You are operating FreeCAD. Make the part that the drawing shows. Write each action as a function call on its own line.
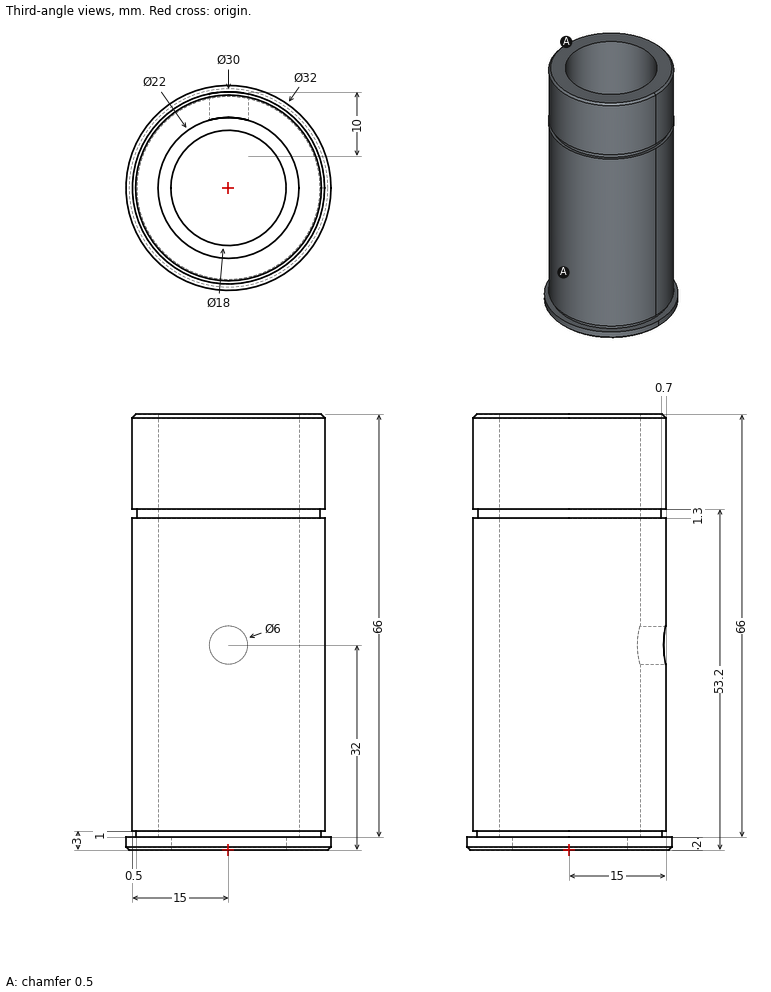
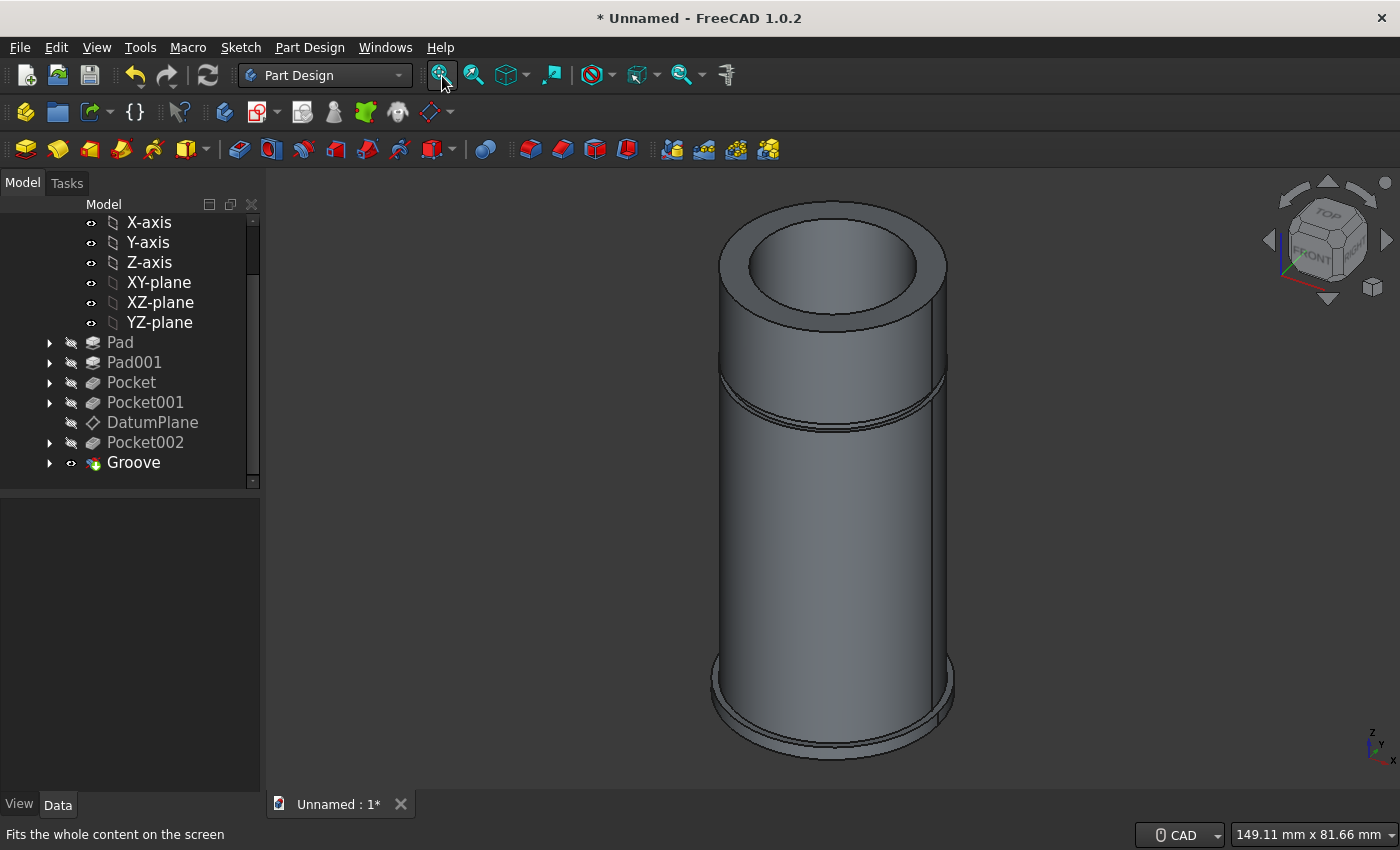
click(719, 272)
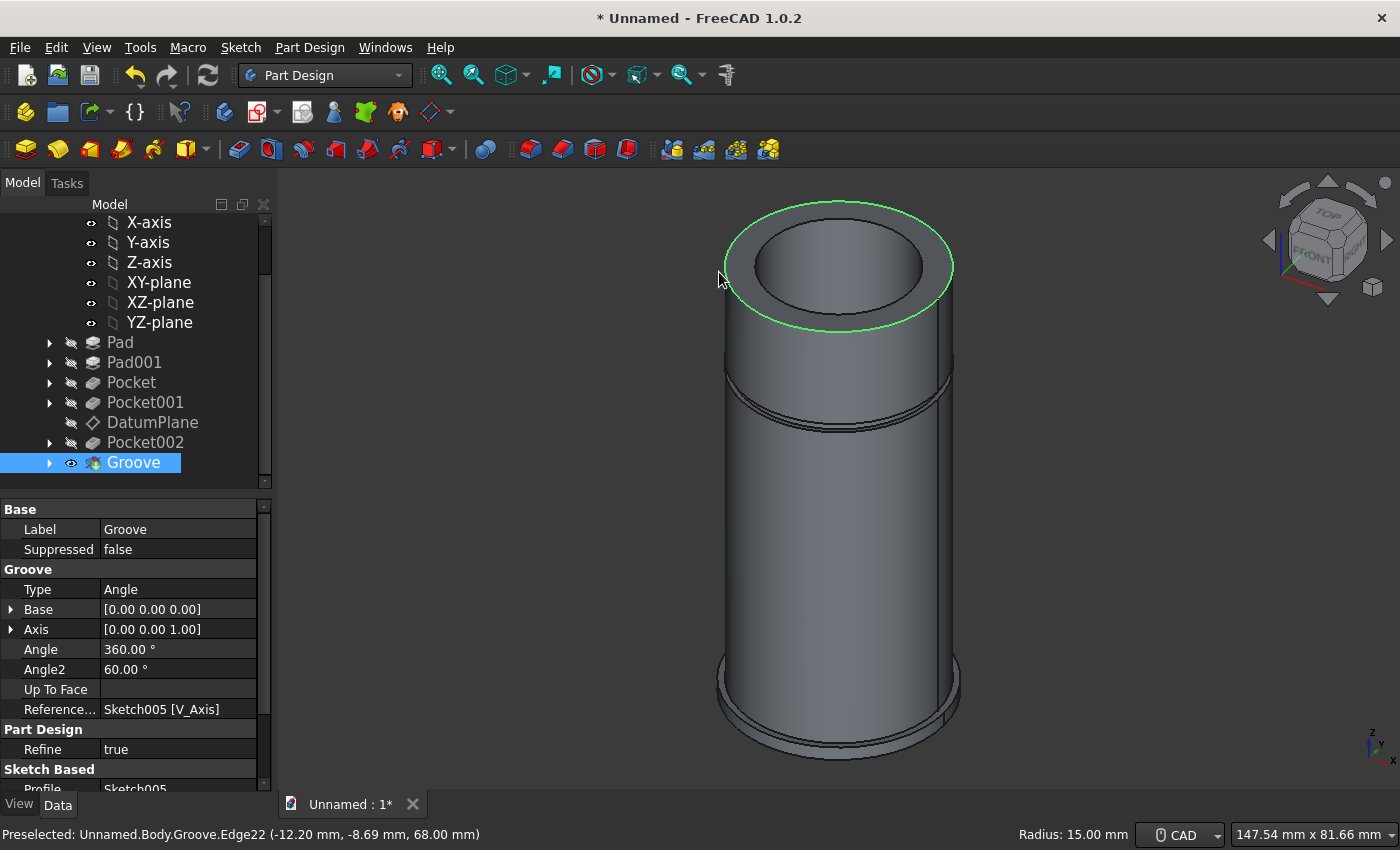
key(0)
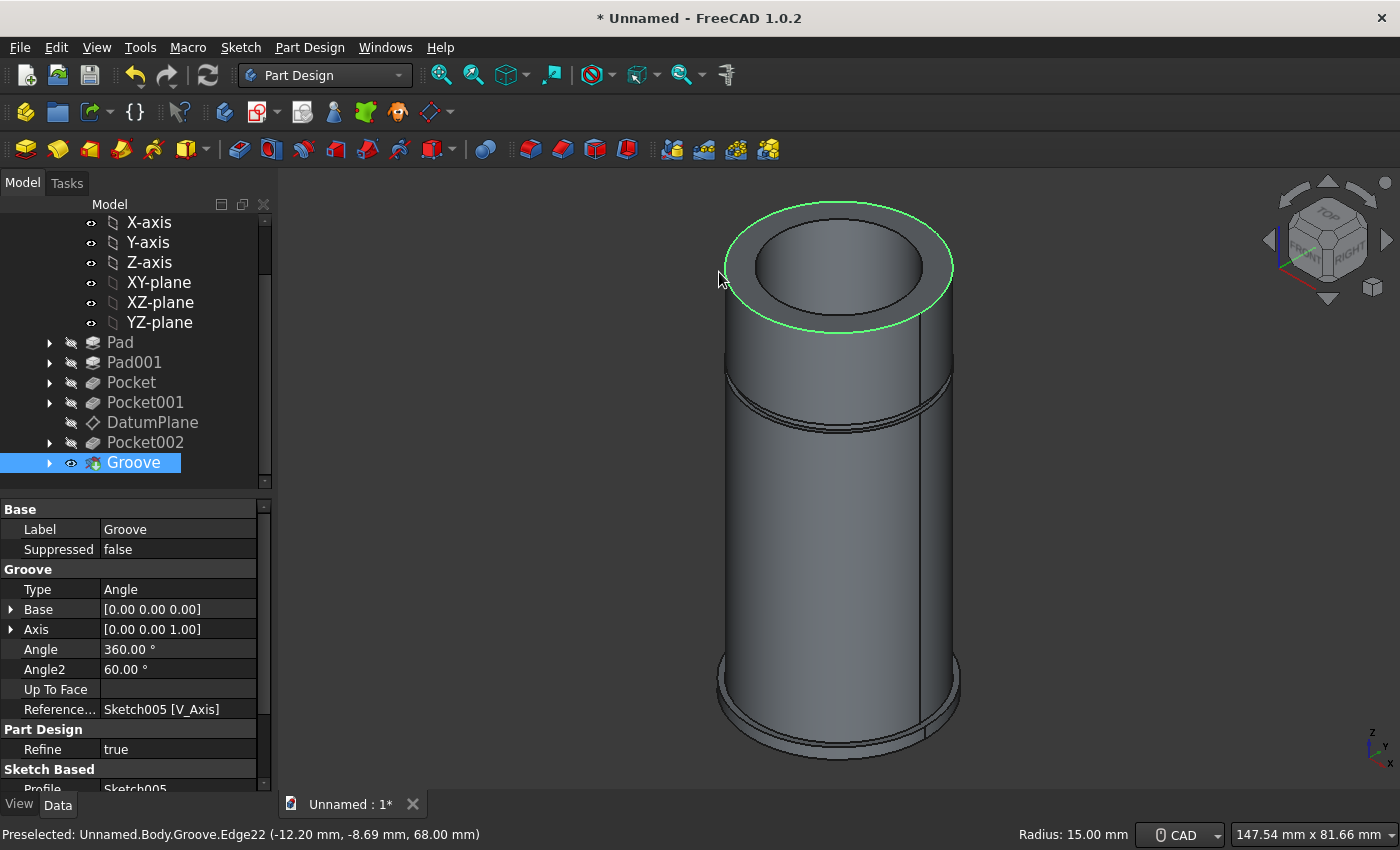
click(442, 76)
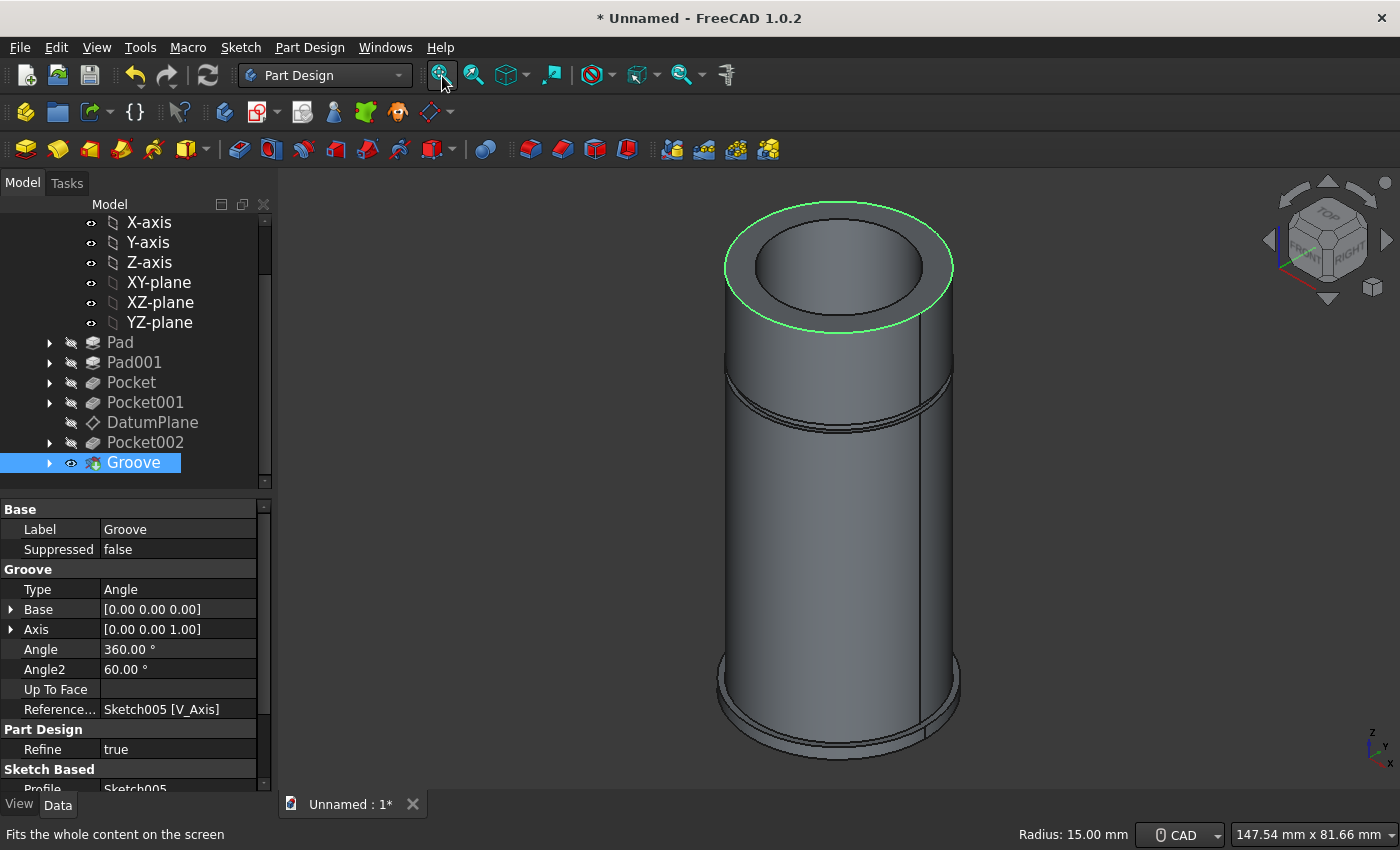
key(2)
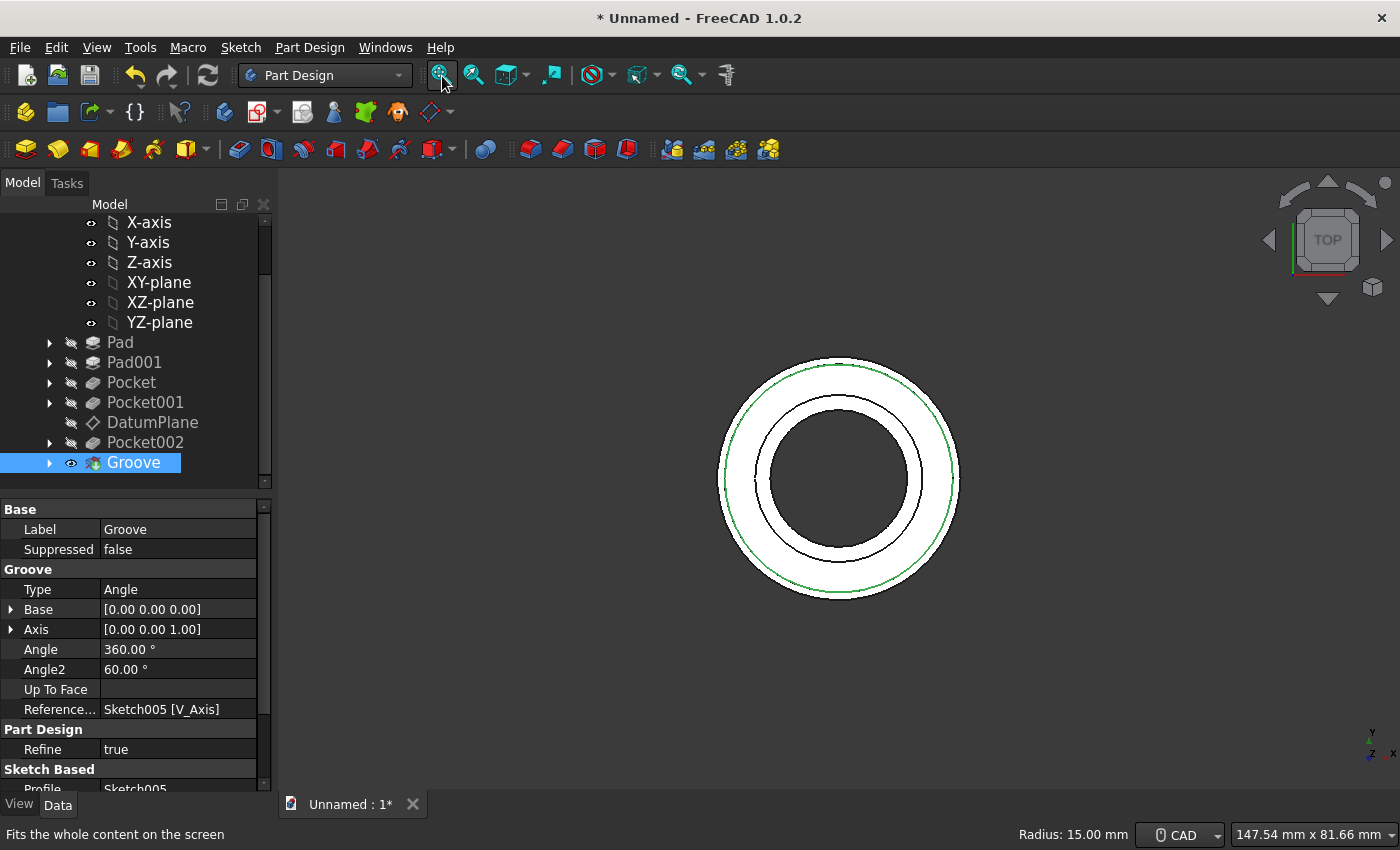
click(442, 76)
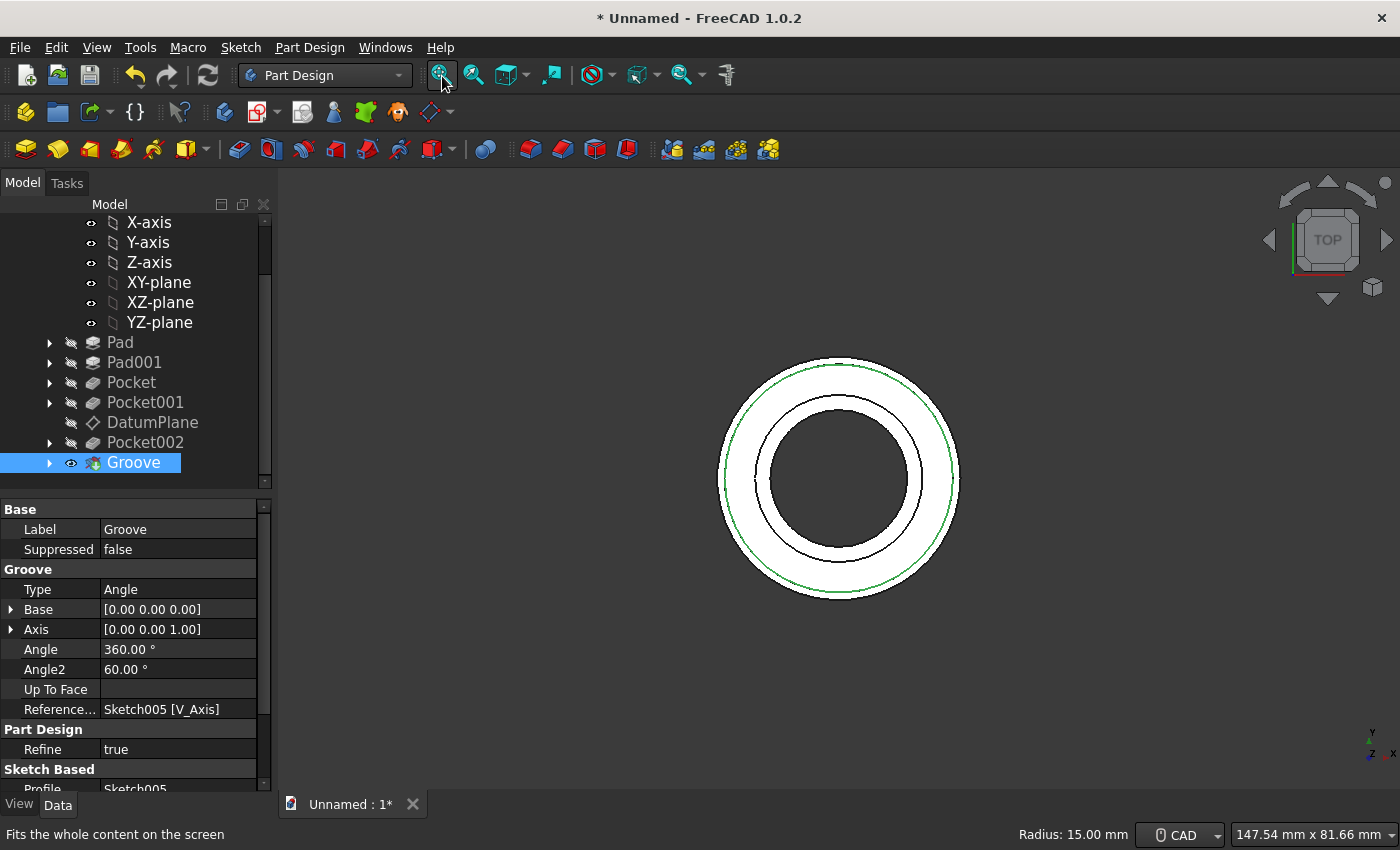
key(1)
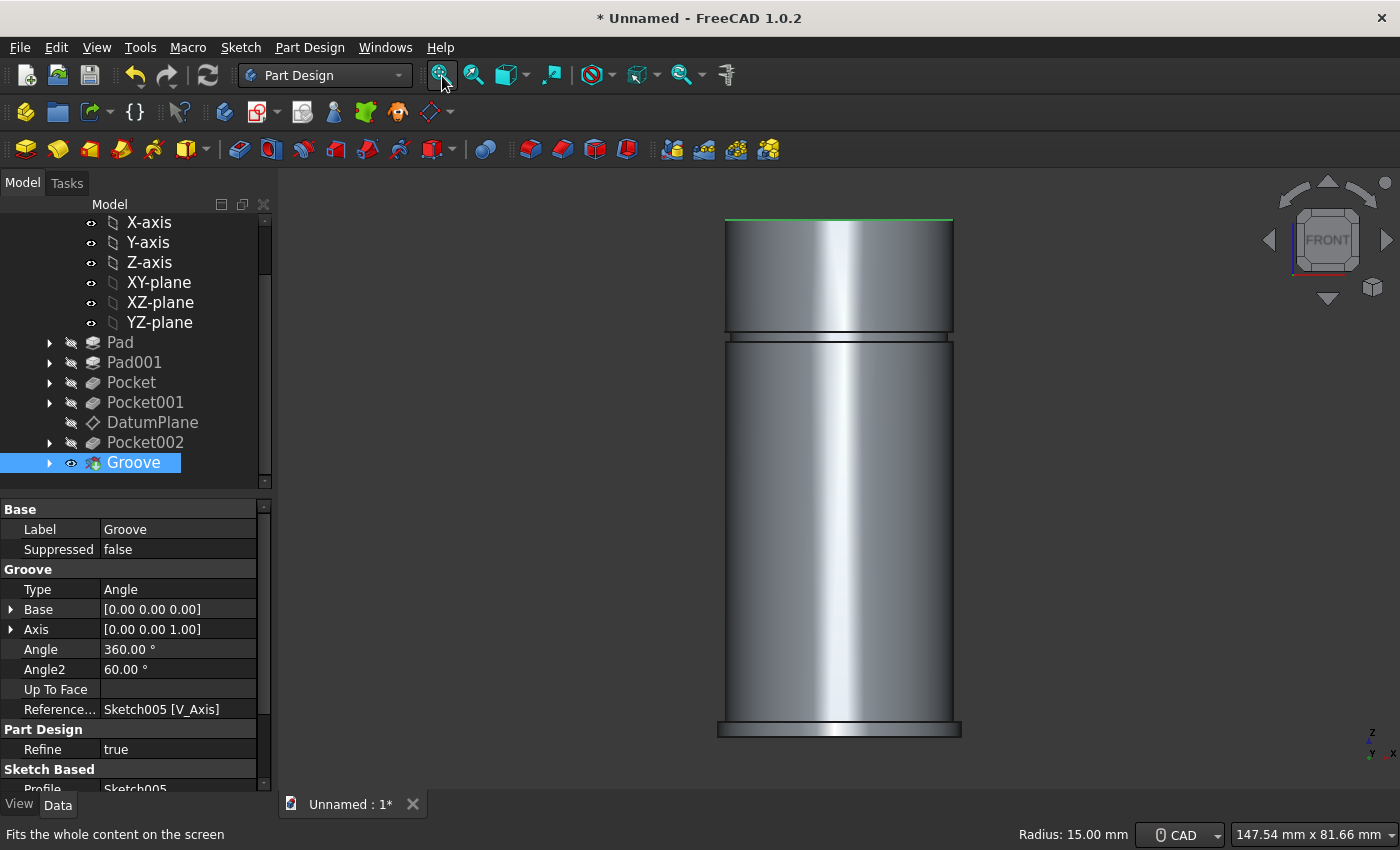
click(740, 736, ctrl)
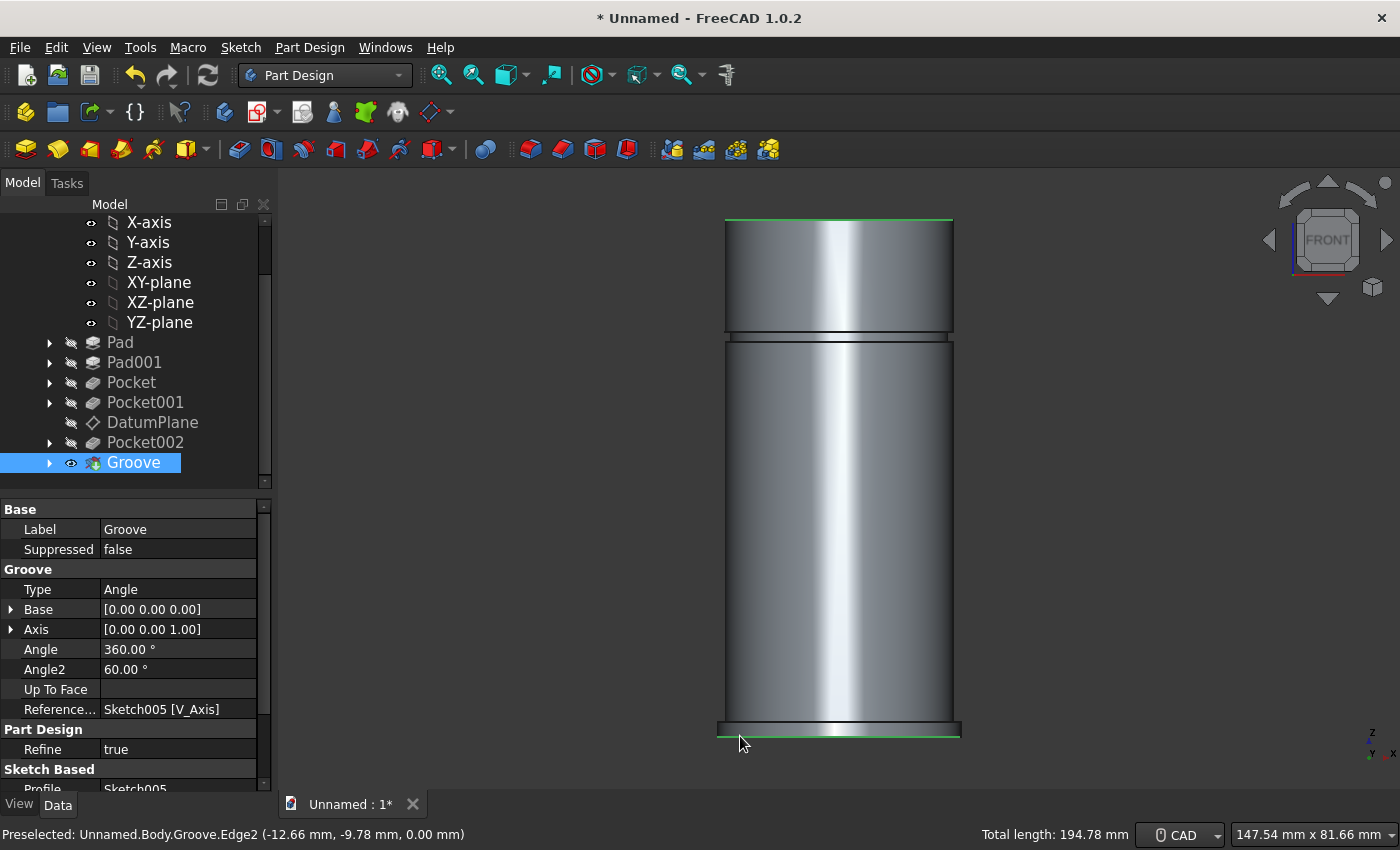
click(564, 150)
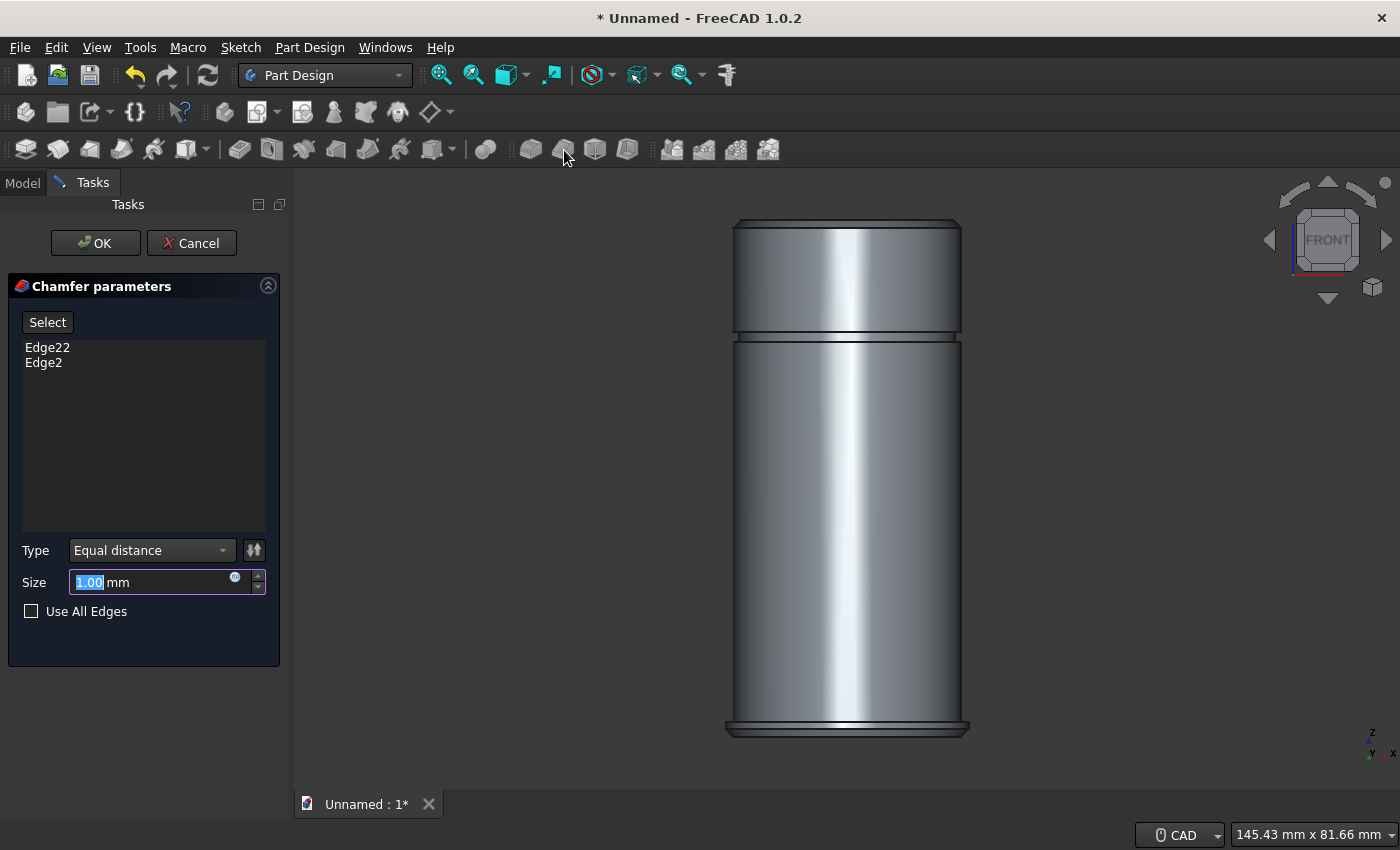
text(0.5)
key(Tab)